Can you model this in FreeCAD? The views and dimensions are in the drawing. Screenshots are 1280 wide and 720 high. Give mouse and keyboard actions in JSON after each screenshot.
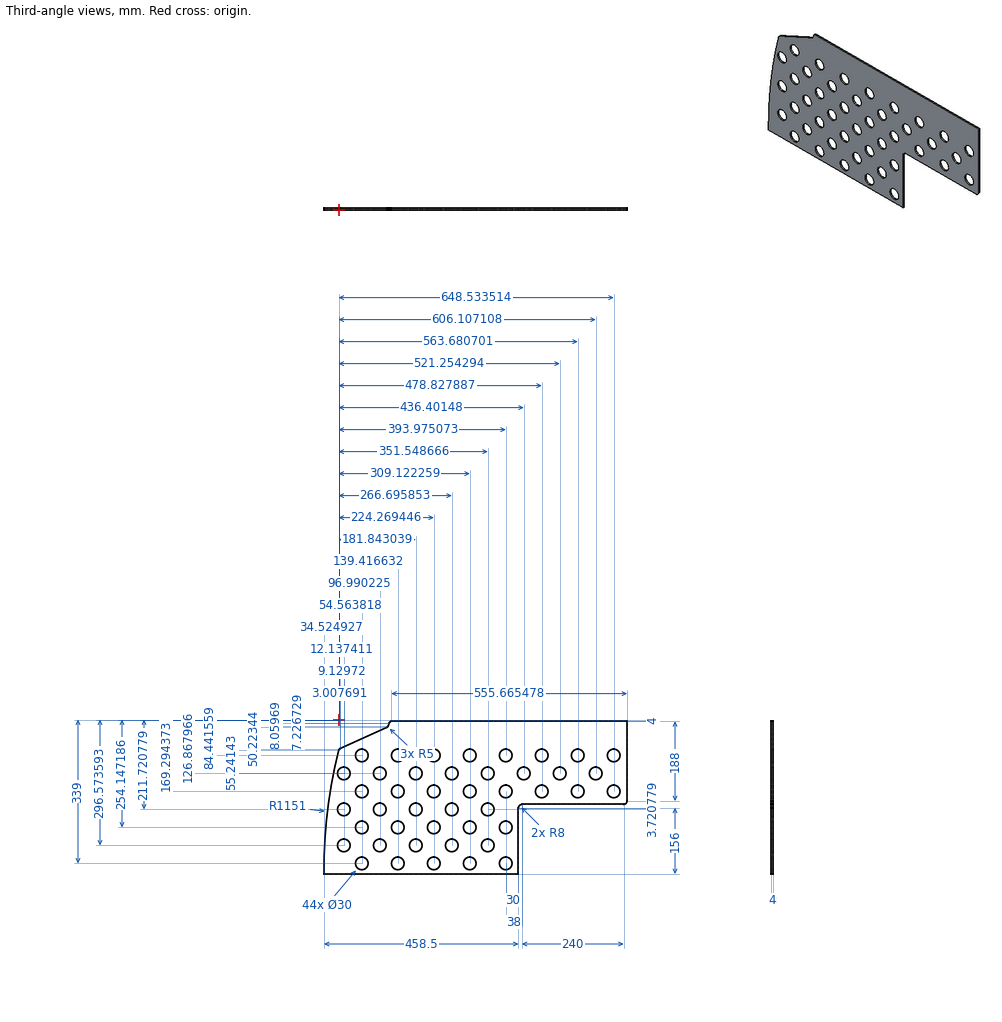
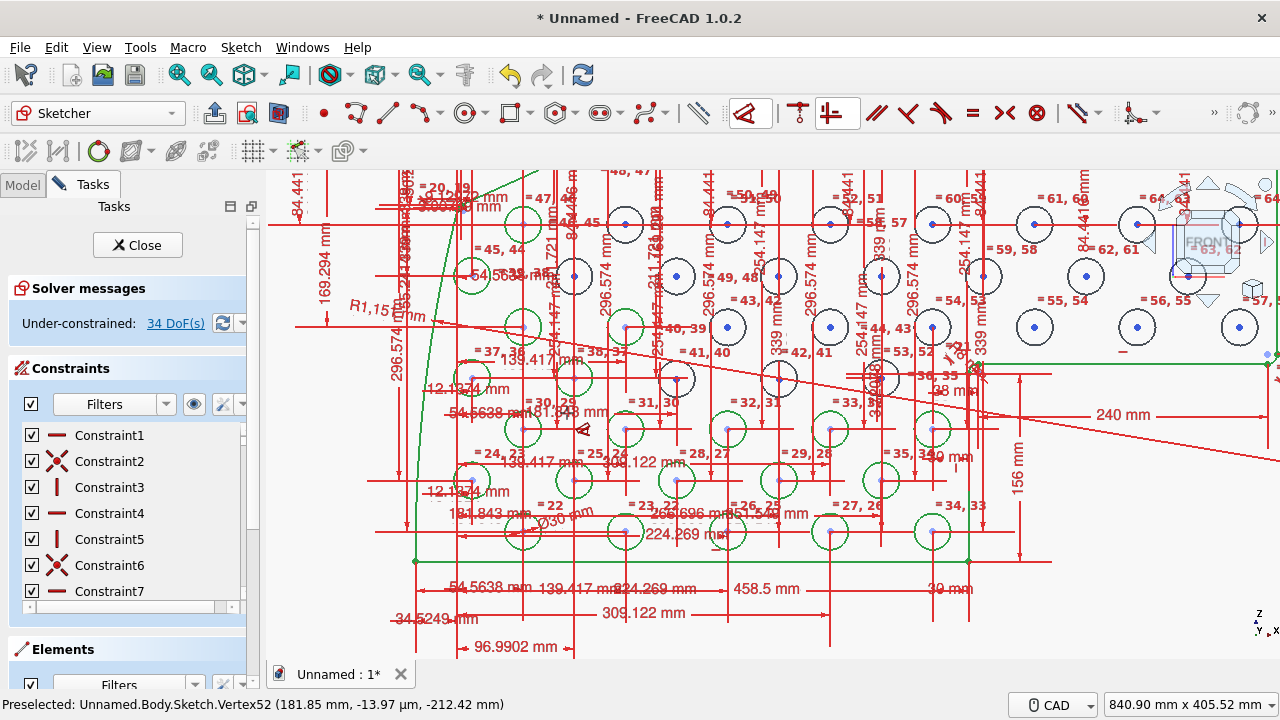
{"action": "left_click", "coordinate": [677, 379]}
{"action": "left_click", "coordinate": [759, 352]}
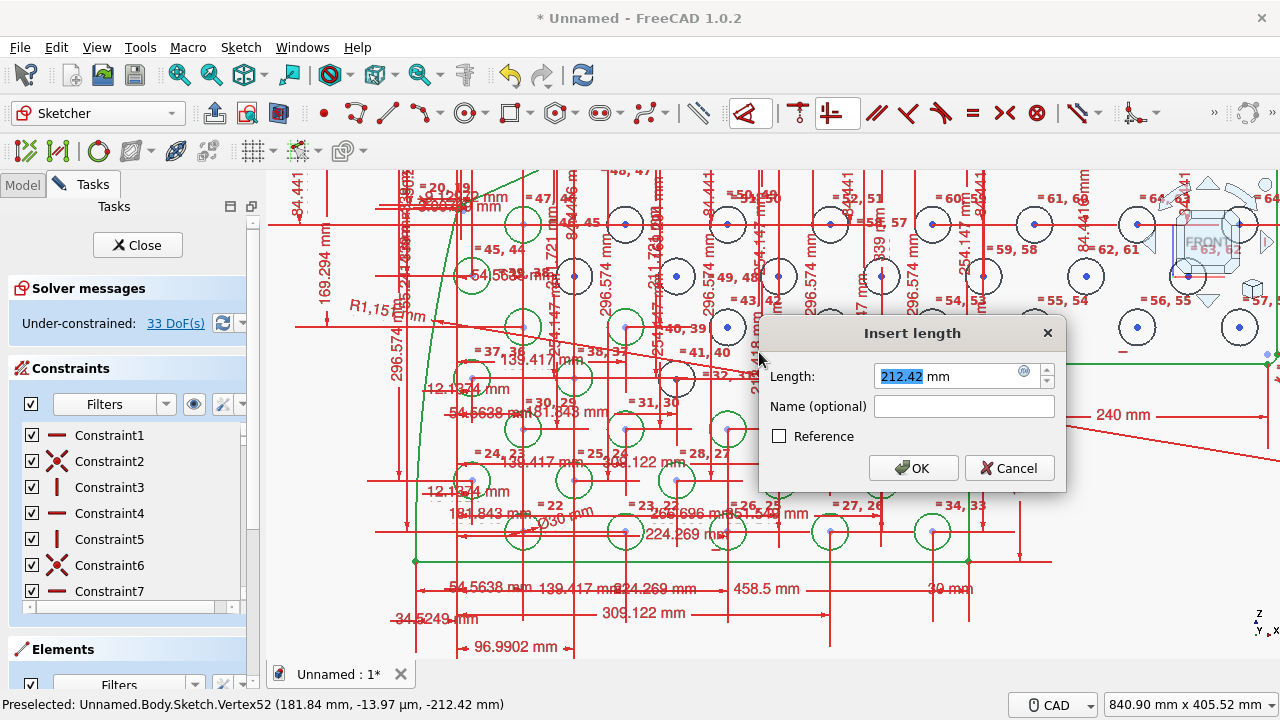
{"action": "type", "text": "211.720779"}
{"action": "key", "text": "Return"}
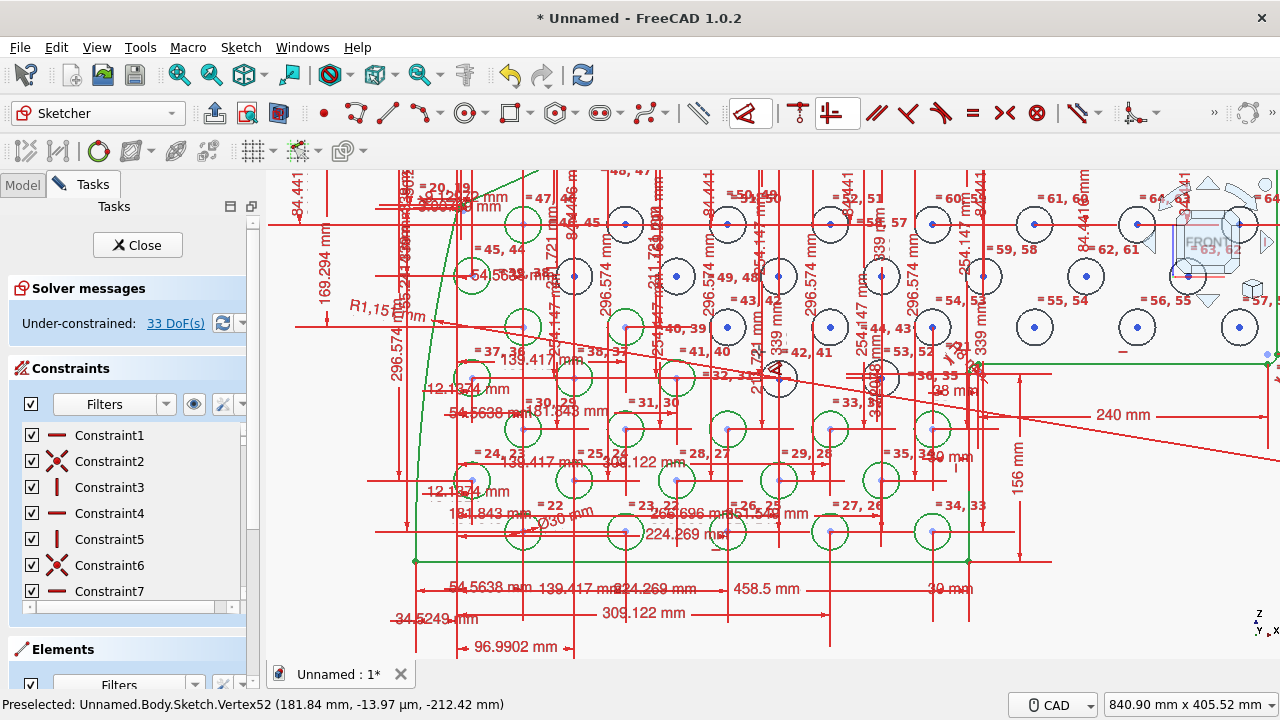
{"action": "left_click", "coordinate": [779, 379]}
{"action": "left_click", "coordinate": [692, 413]}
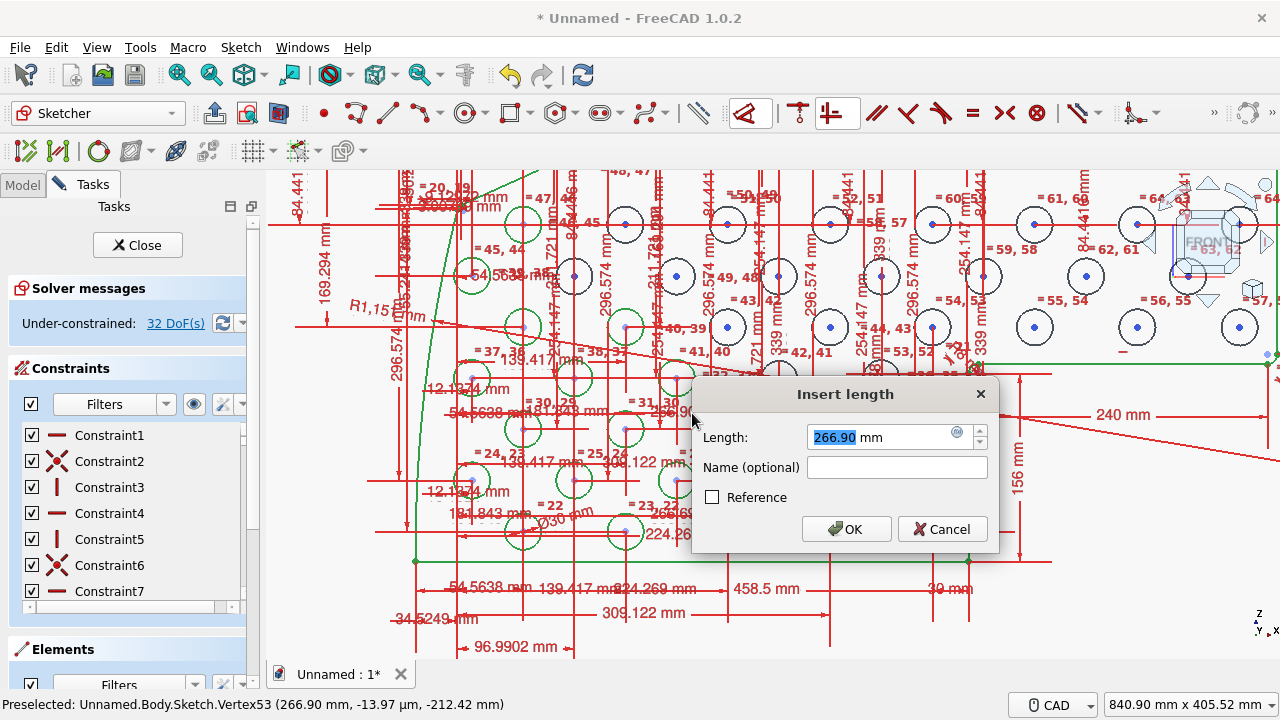
{"action": "type", "text": "266.695853"}
{"action": "key", "text": "Return"}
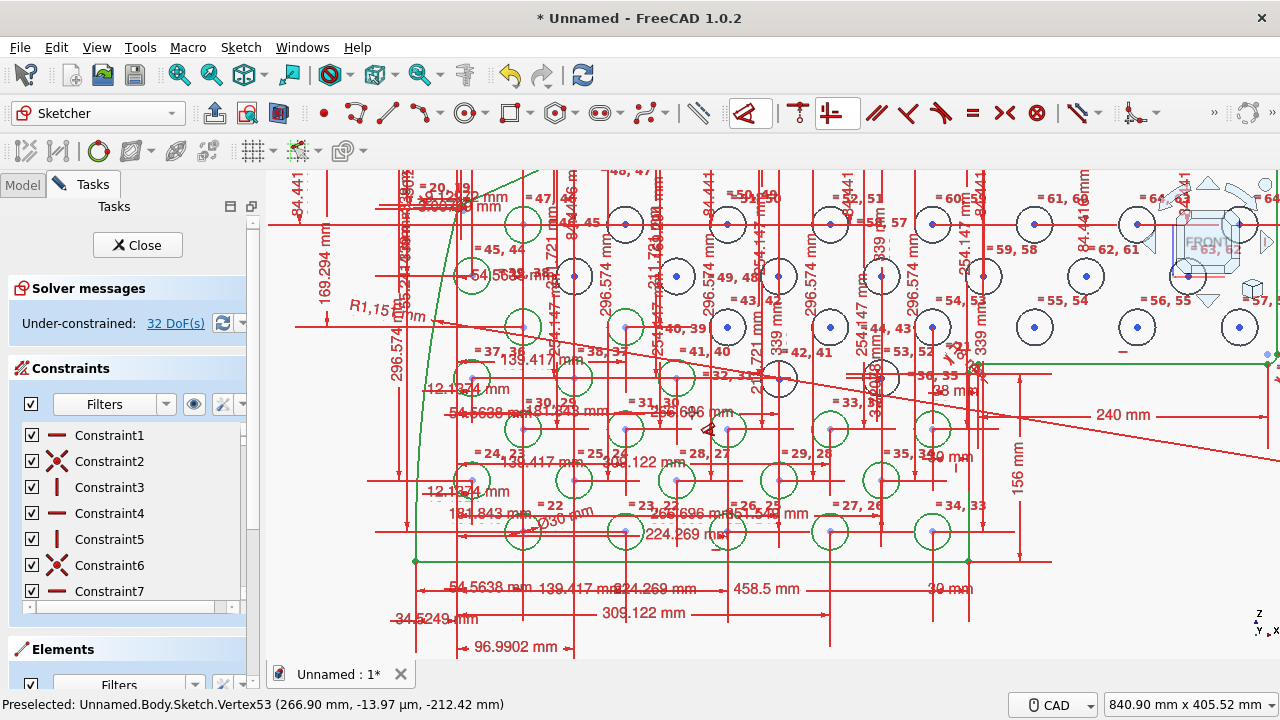
{"action": "left_click", "coordinate": [779, 379]}
{"action": "left_click", "coordinate": [861, 352]}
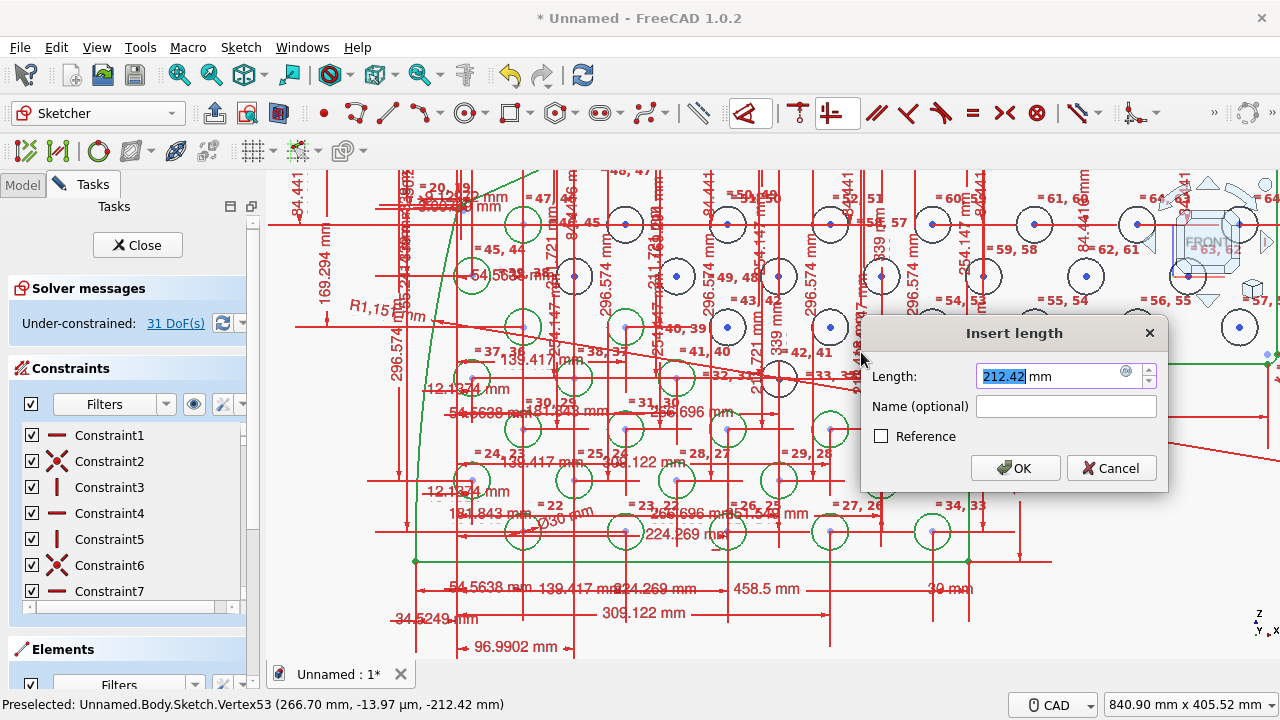
{"action": "type", "text": "211.720779"}
{"action": "key", "text": "Return"}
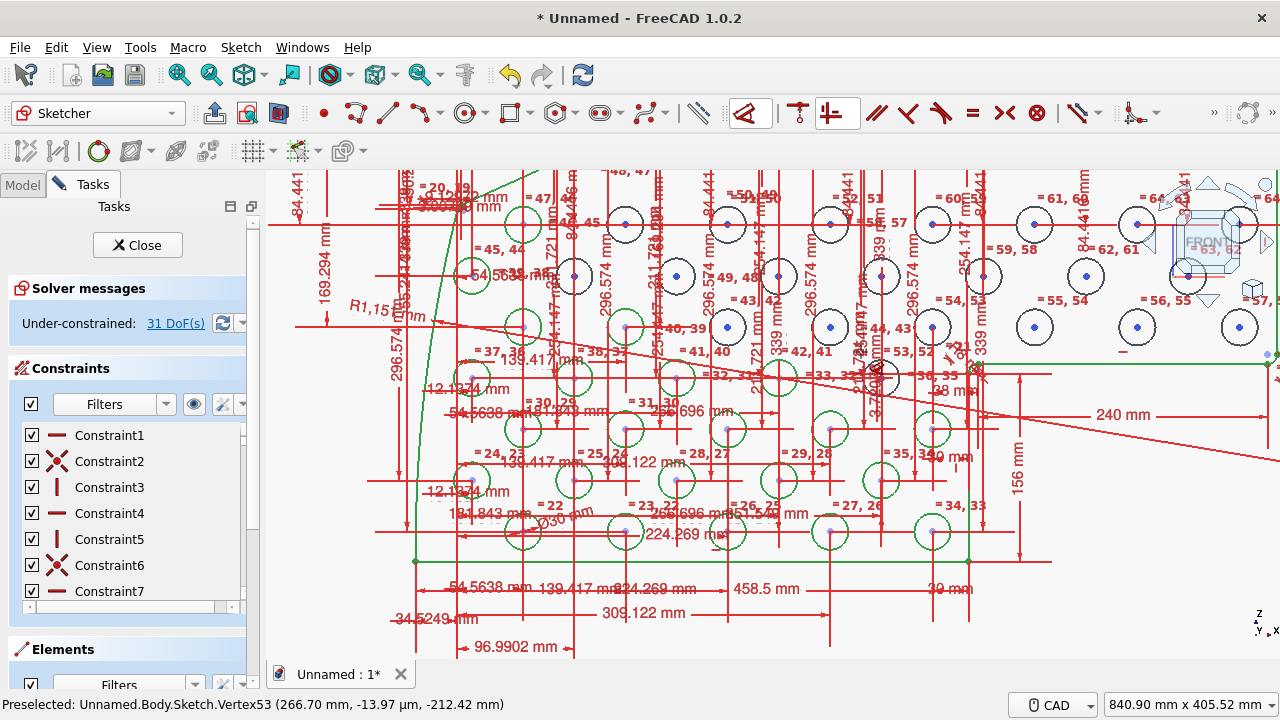
{"action": "left_click", "coordinate": [728, 327]}
{"action": "left_click", "coordinate": [593, 433]}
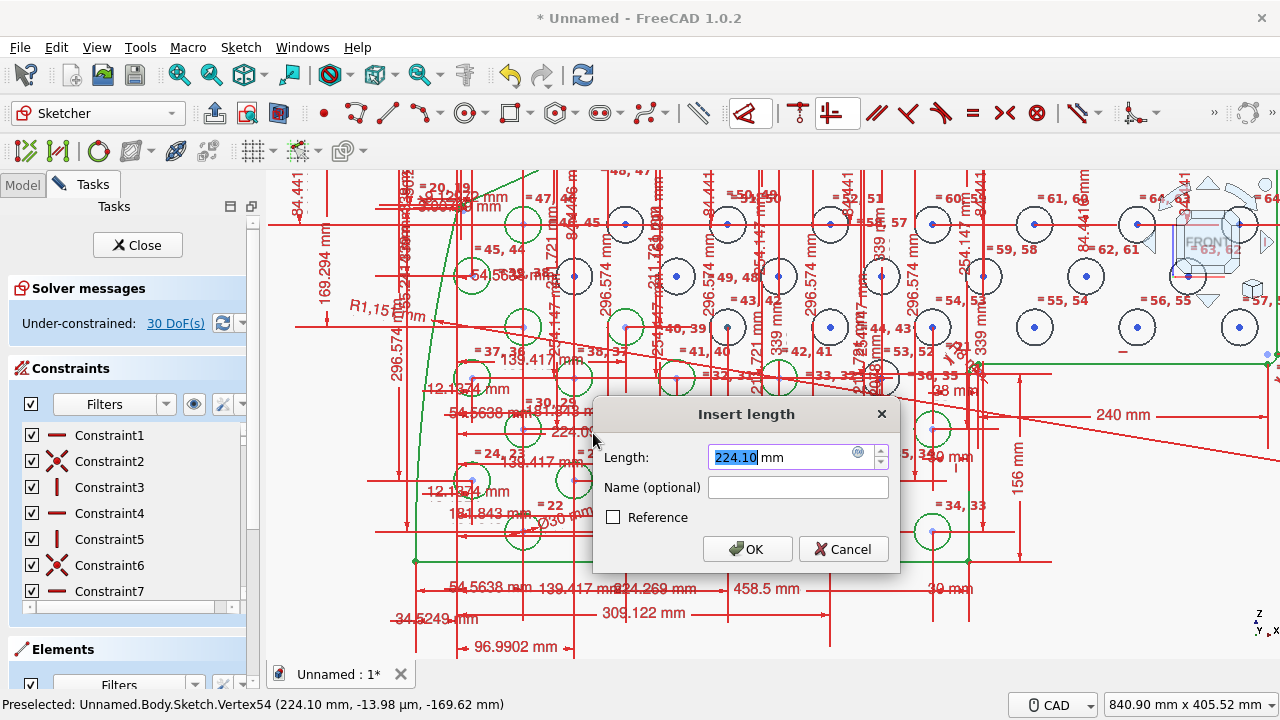
{"action": "type", "text": "224.269446"}
{"action": "key", "text": "Return"}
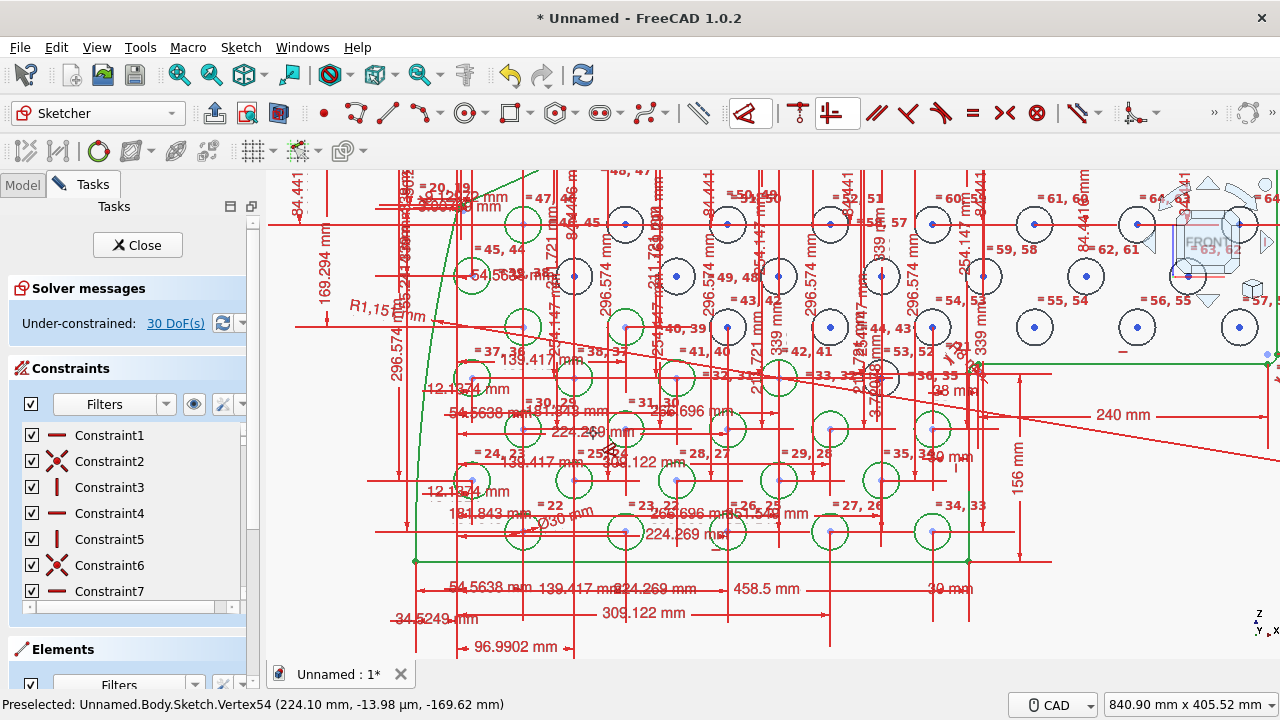
{"action": "left_click", "coordinate": [728, 327]}
{"action": "left_click", "coordinate": [327, 233]}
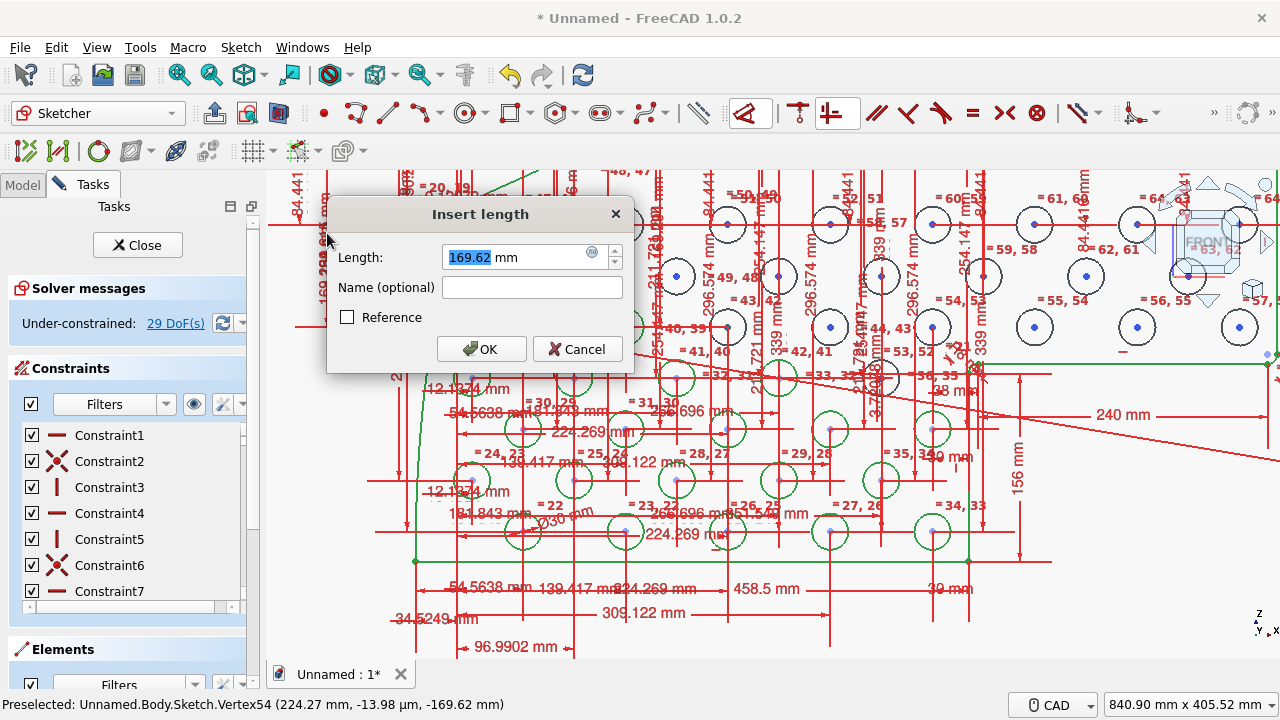
{"action": "type", "text": "169.294373"}
{"action": "key", "text": "Return"}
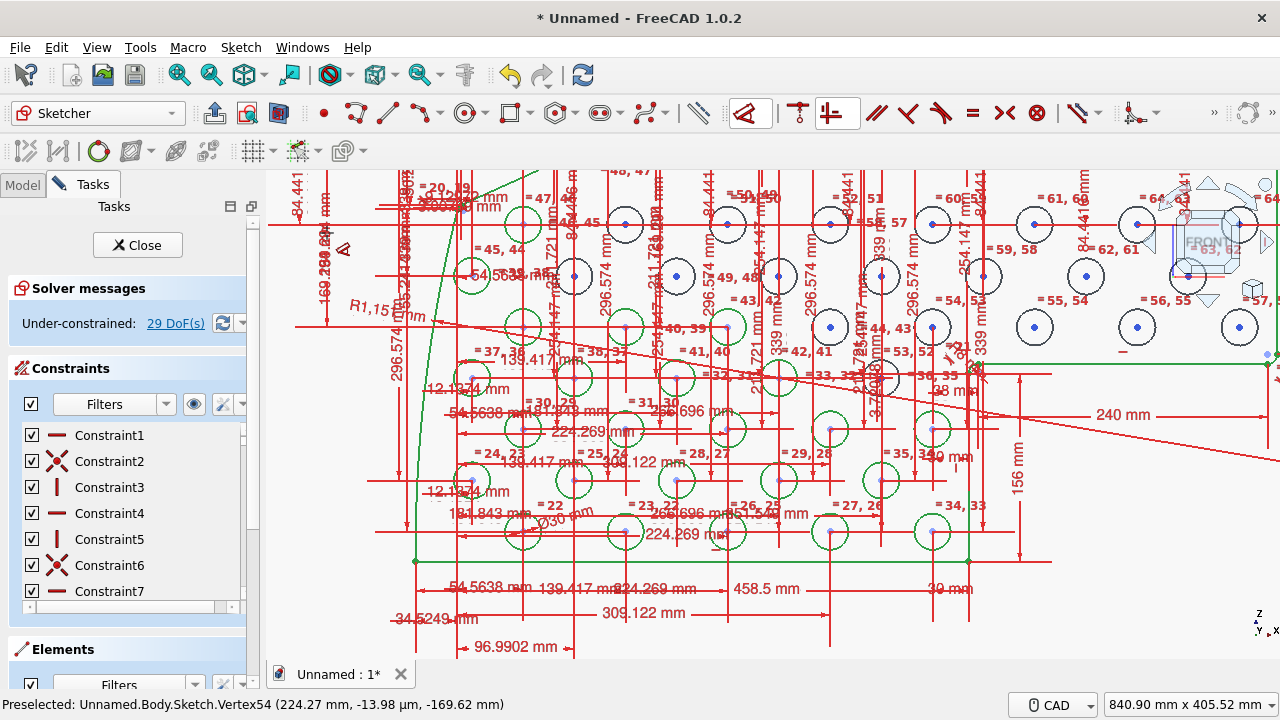
{"action": "left_click", "coordinate": [830, 327]}
{"action": "left_click", "coordinate": [644, 361]}